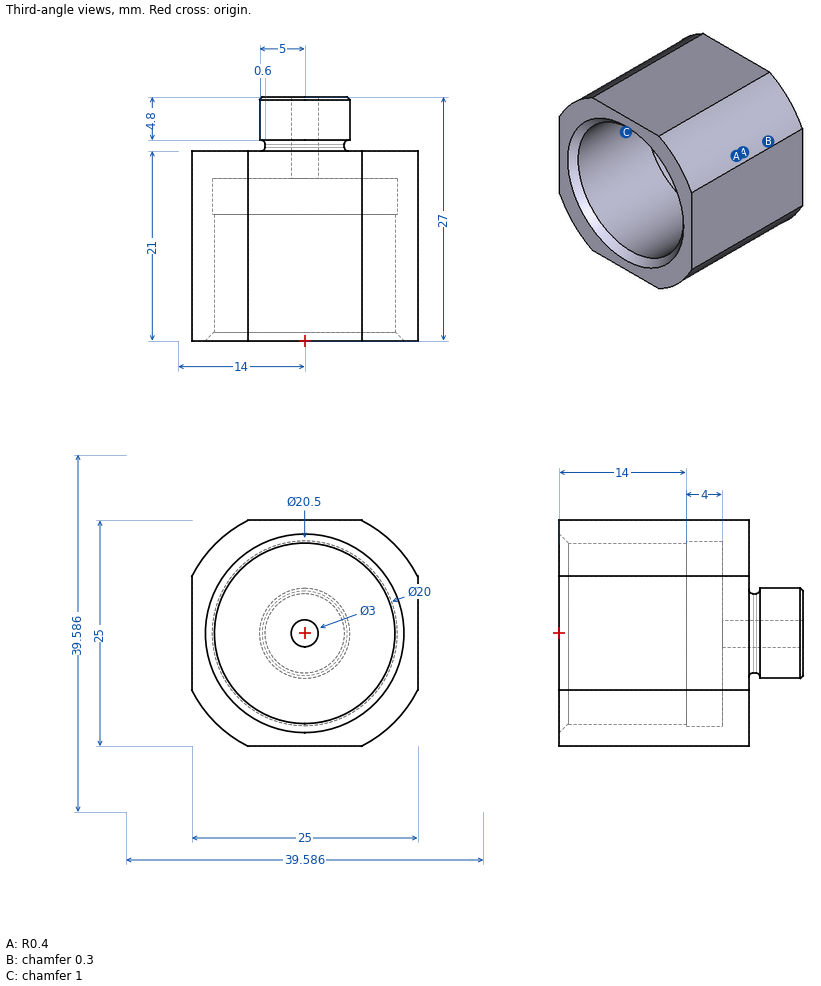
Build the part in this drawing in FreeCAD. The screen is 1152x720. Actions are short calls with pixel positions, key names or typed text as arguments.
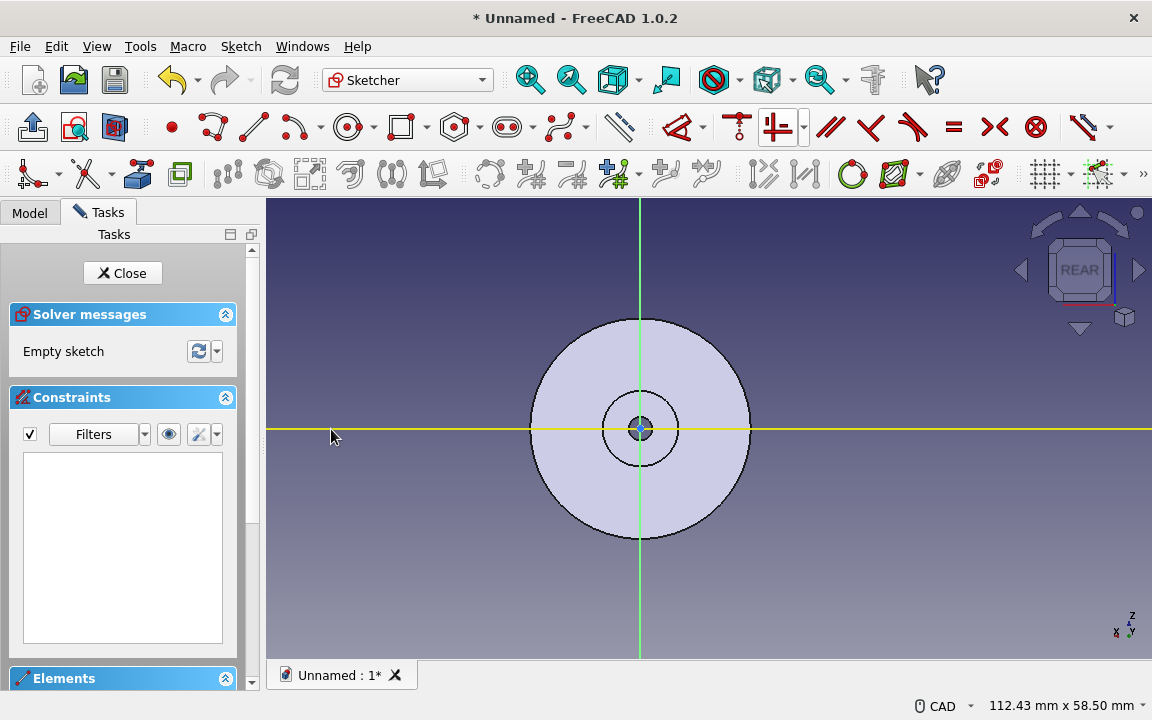
key(g)
key(v)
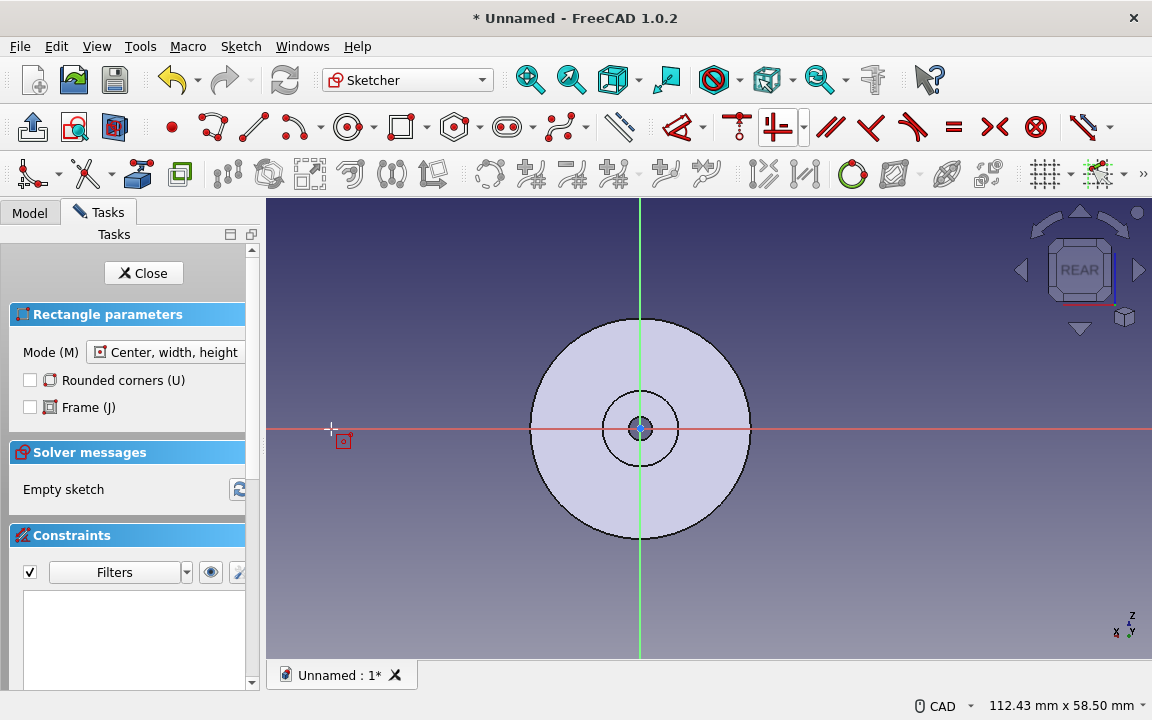
click(640, 429)
click(796, 273)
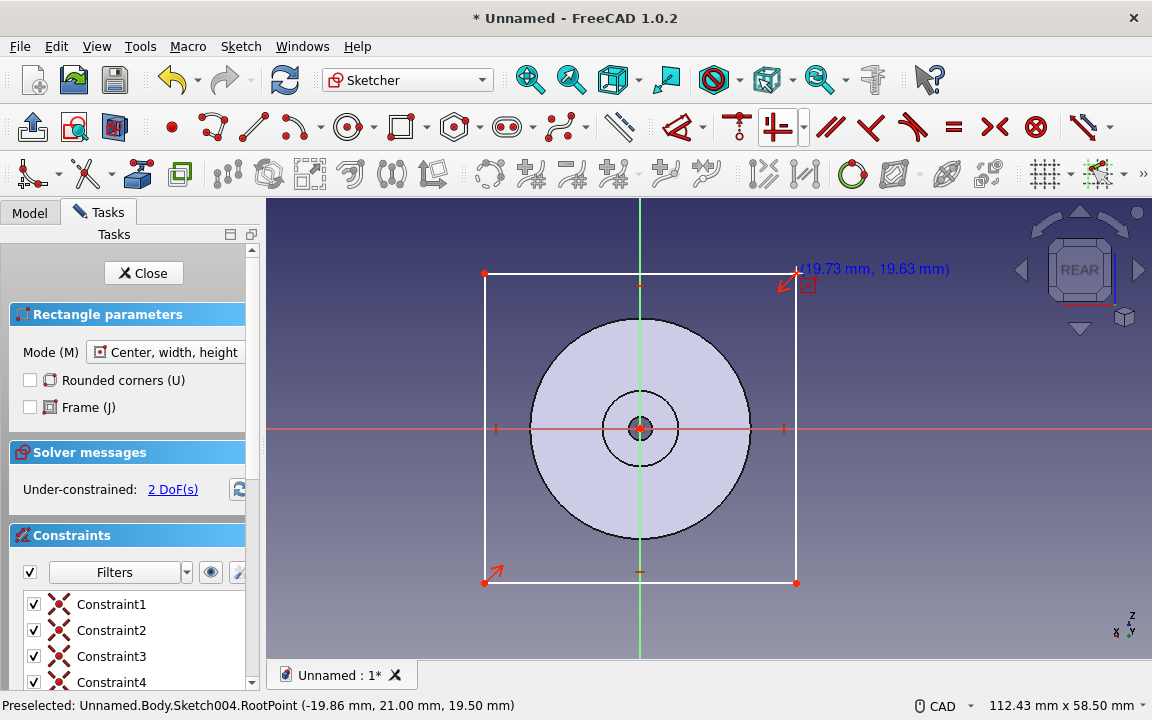
click(640, 429)
click(739, 330)
key(Escape)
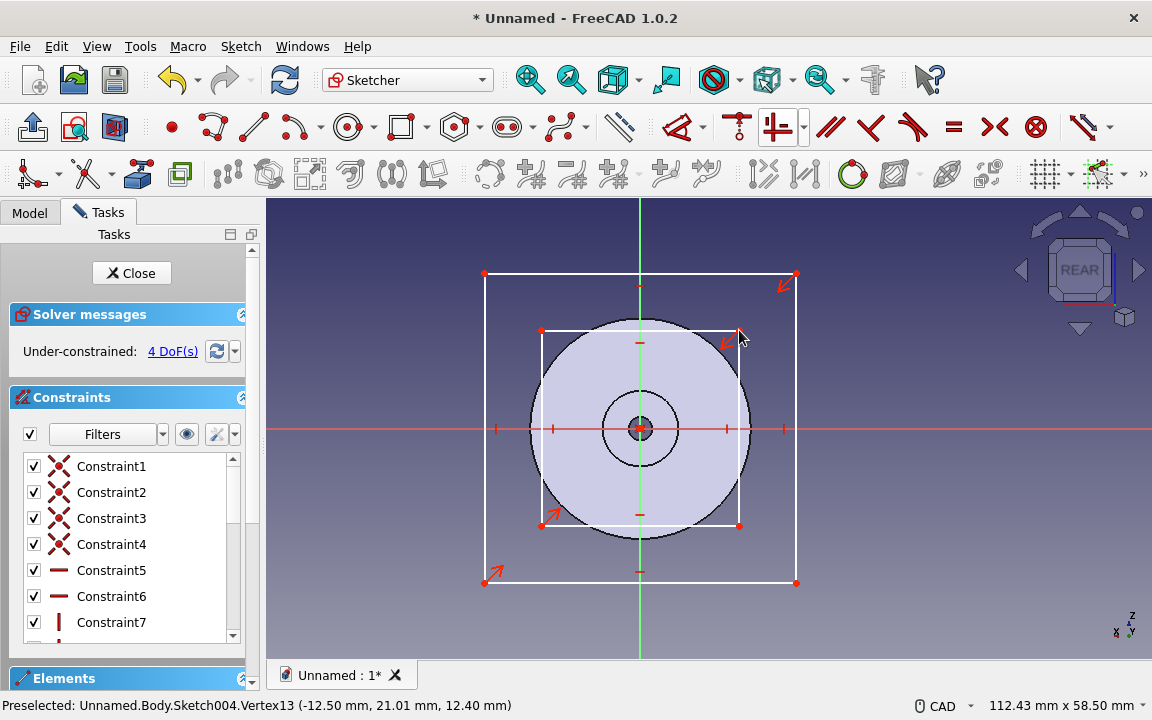
click(676, 128)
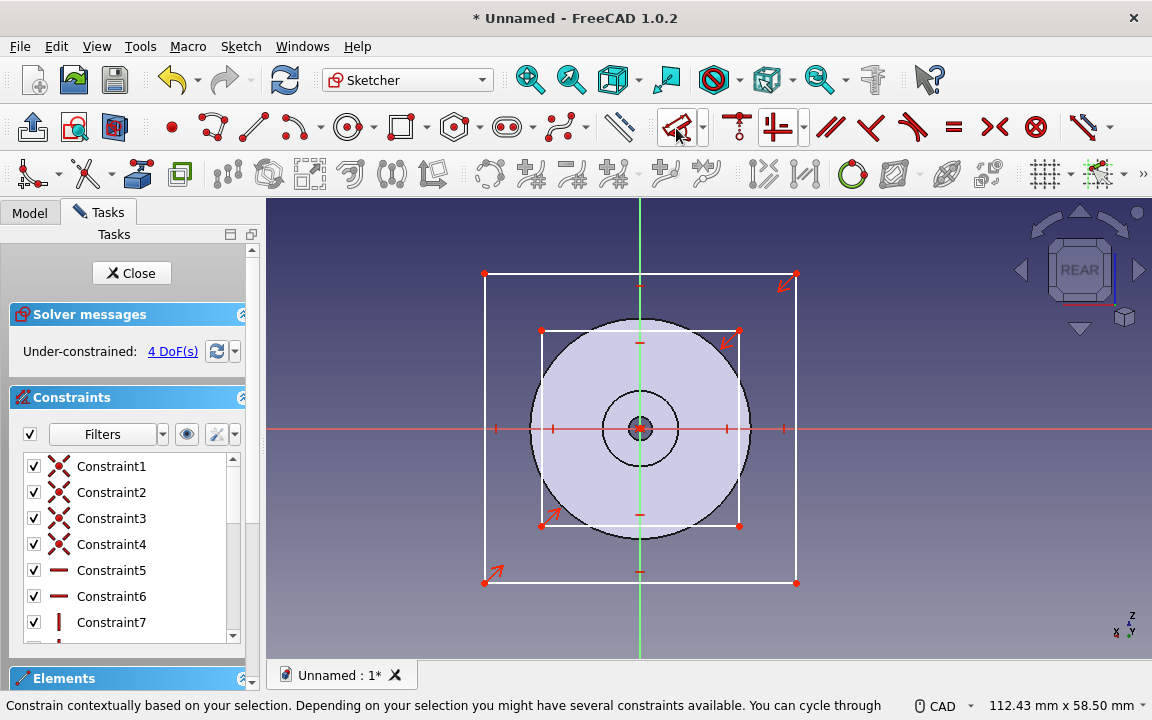
click(601, 526)
click(595, 560)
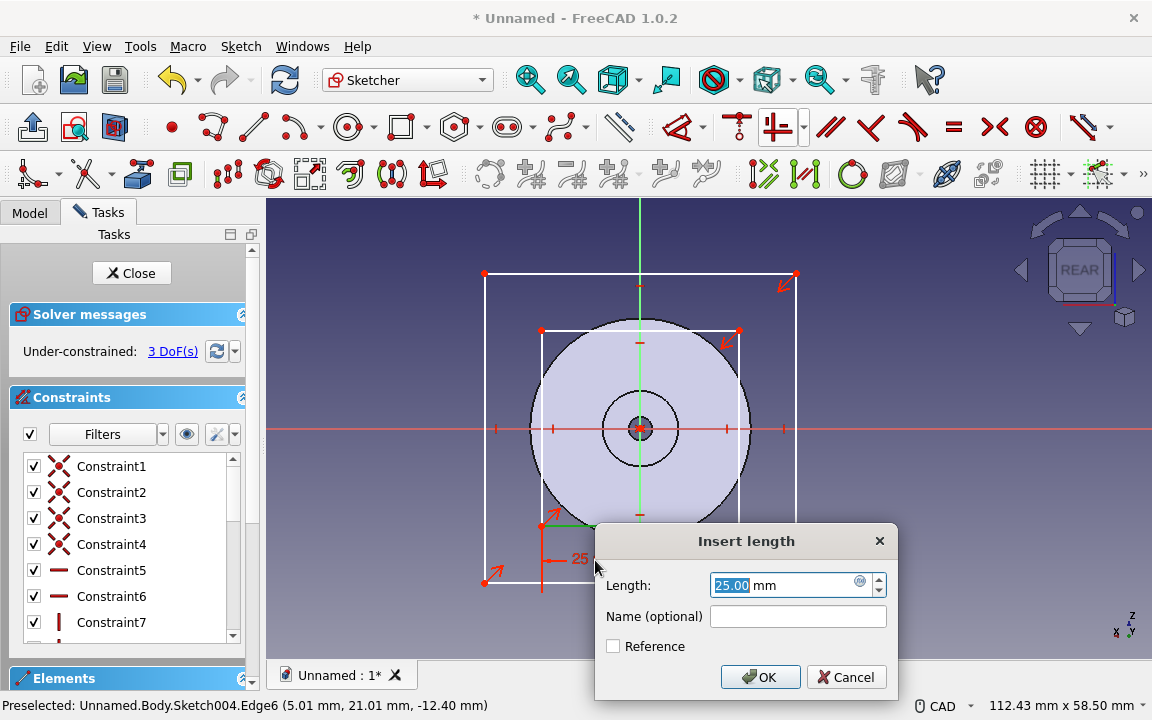
text(25)
key(Return)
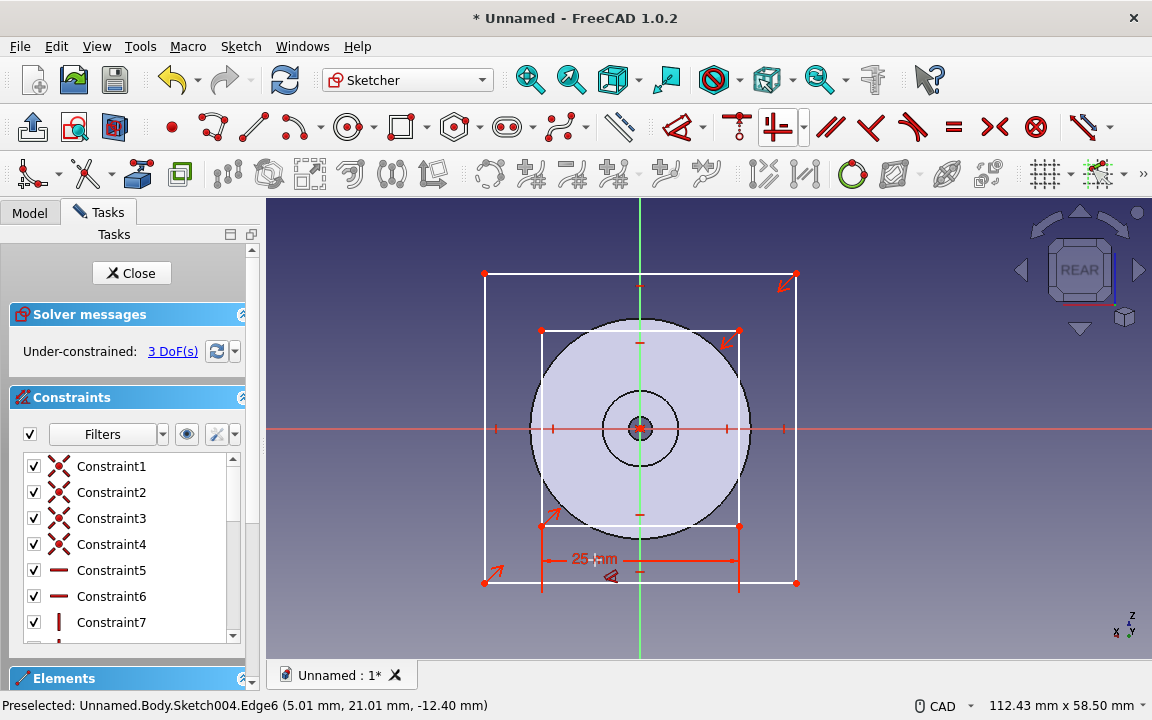
click(739, 468)
click(773, 384)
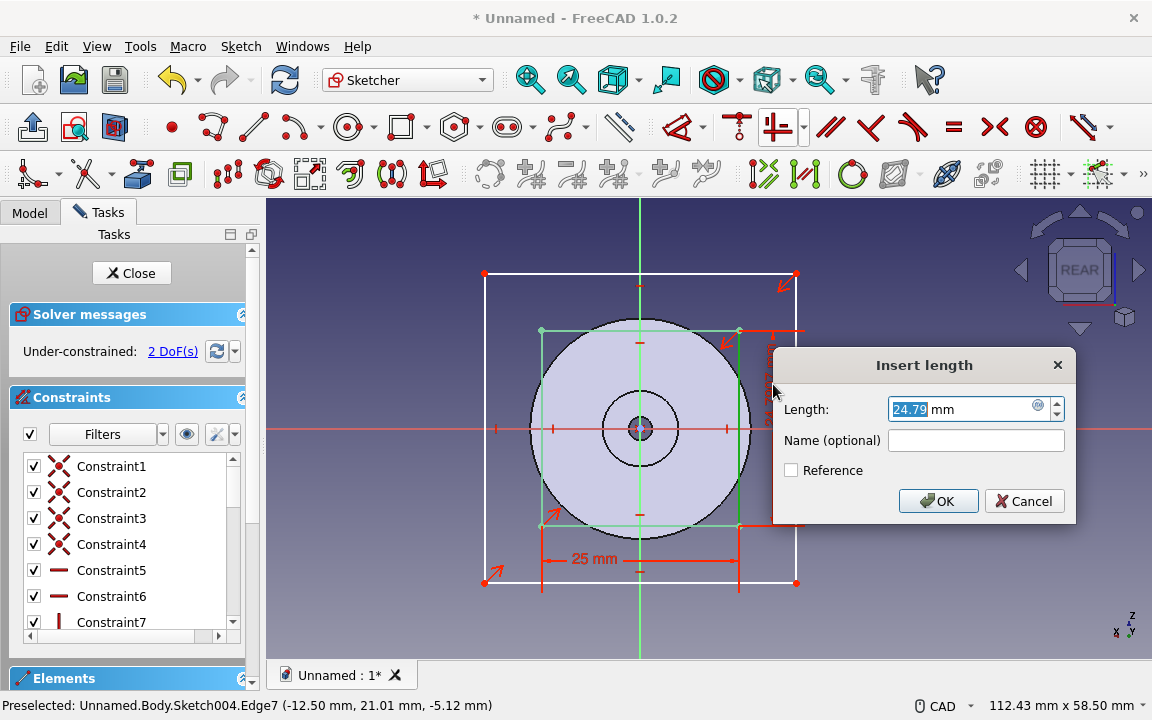
text(25)
key(Return)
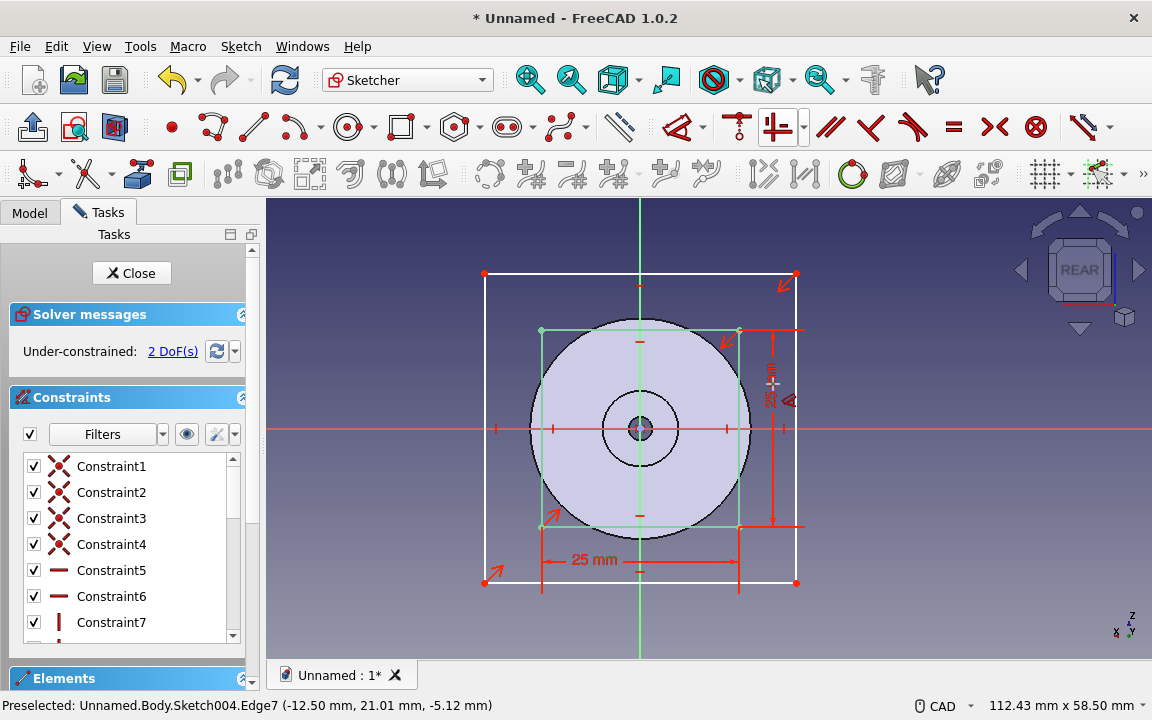
click(578, 583)
click(569, 617)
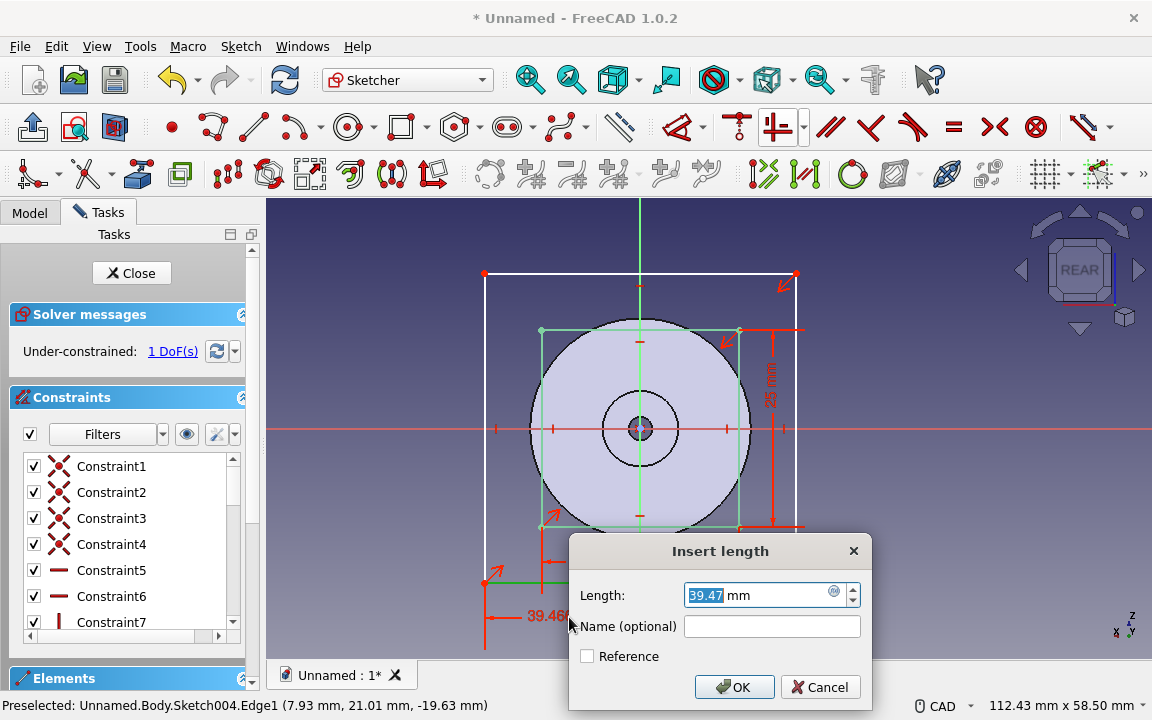
text(39.586)
key(Return)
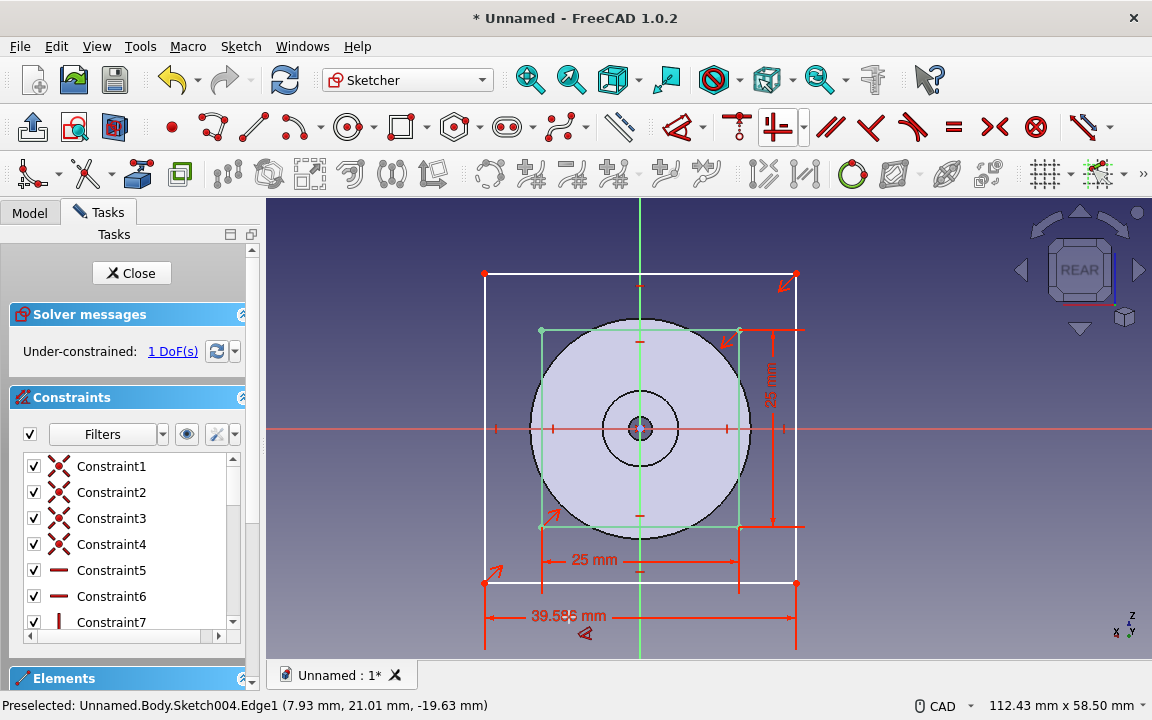
click(796, 491)
click(830, 358)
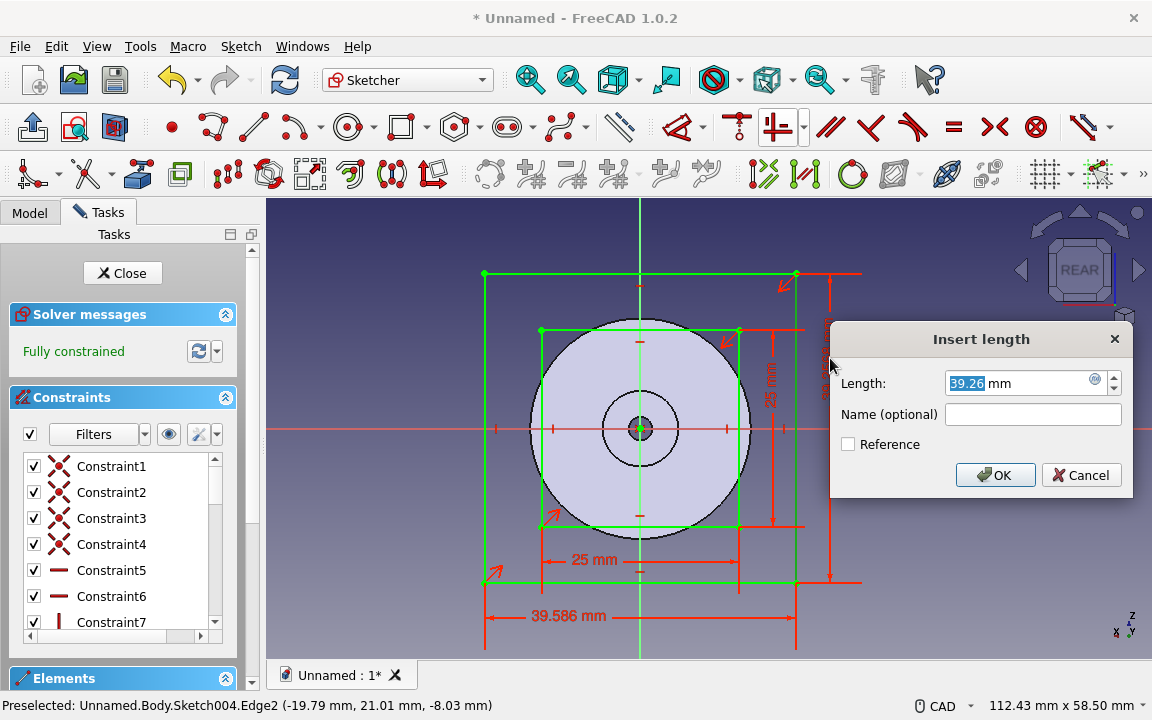
text(39.586)
key(Return)
key(Escape)